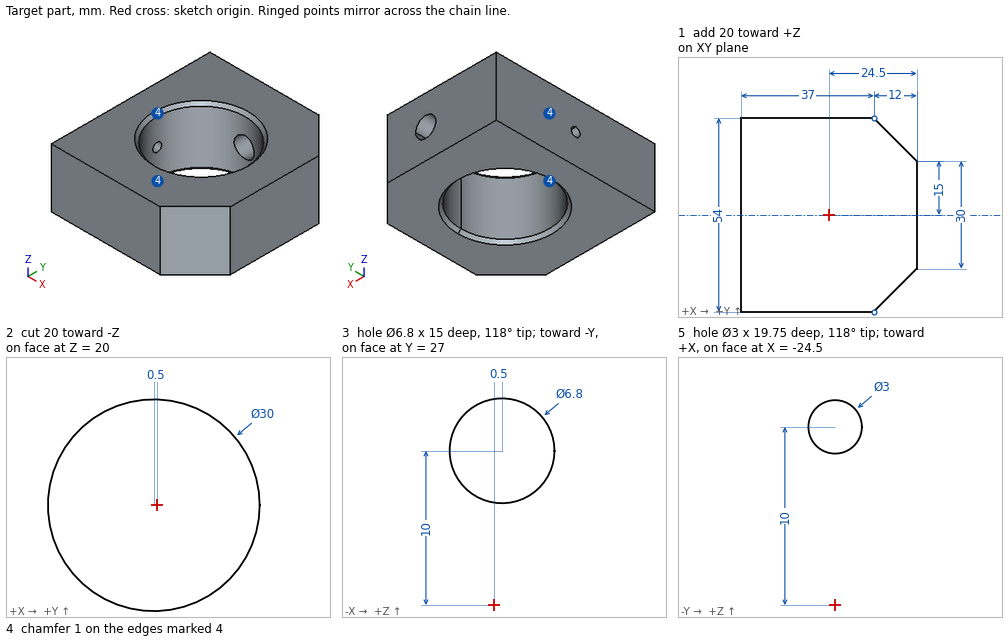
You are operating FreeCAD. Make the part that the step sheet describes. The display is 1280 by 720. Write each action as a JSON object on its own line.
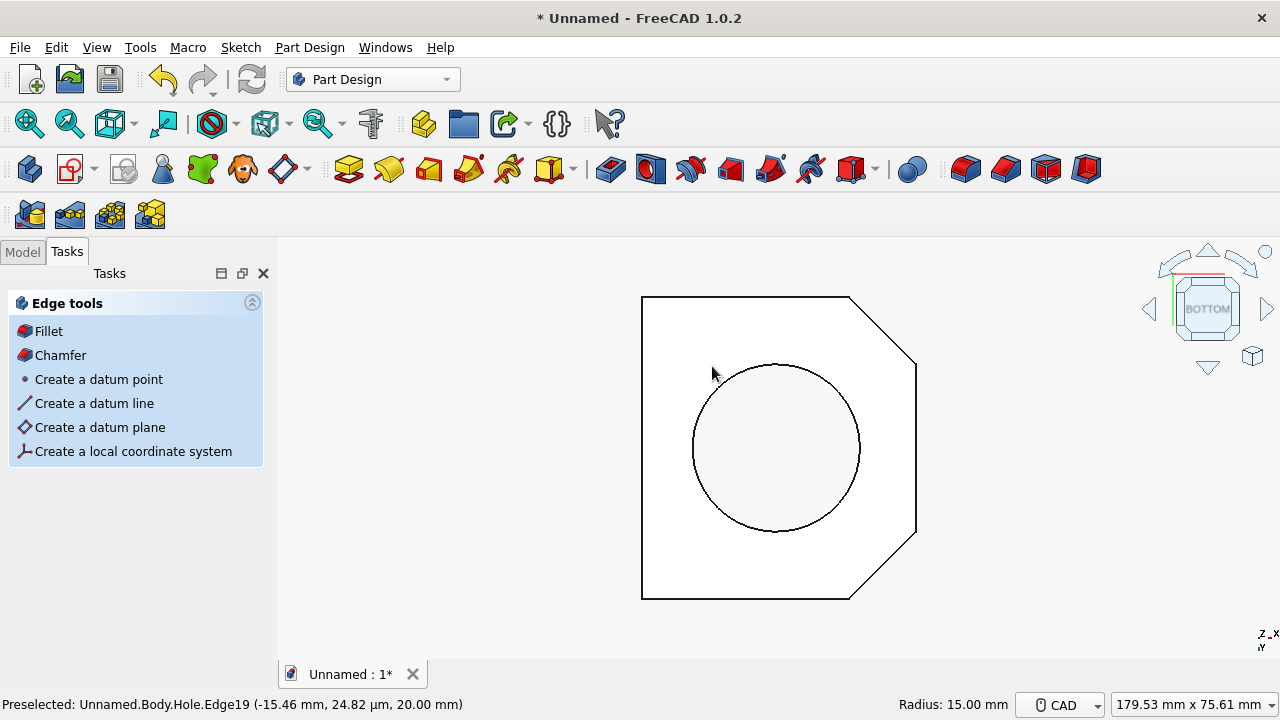
{"action": "left_click", "coordinate": [708, 496], "text": "ctrl"}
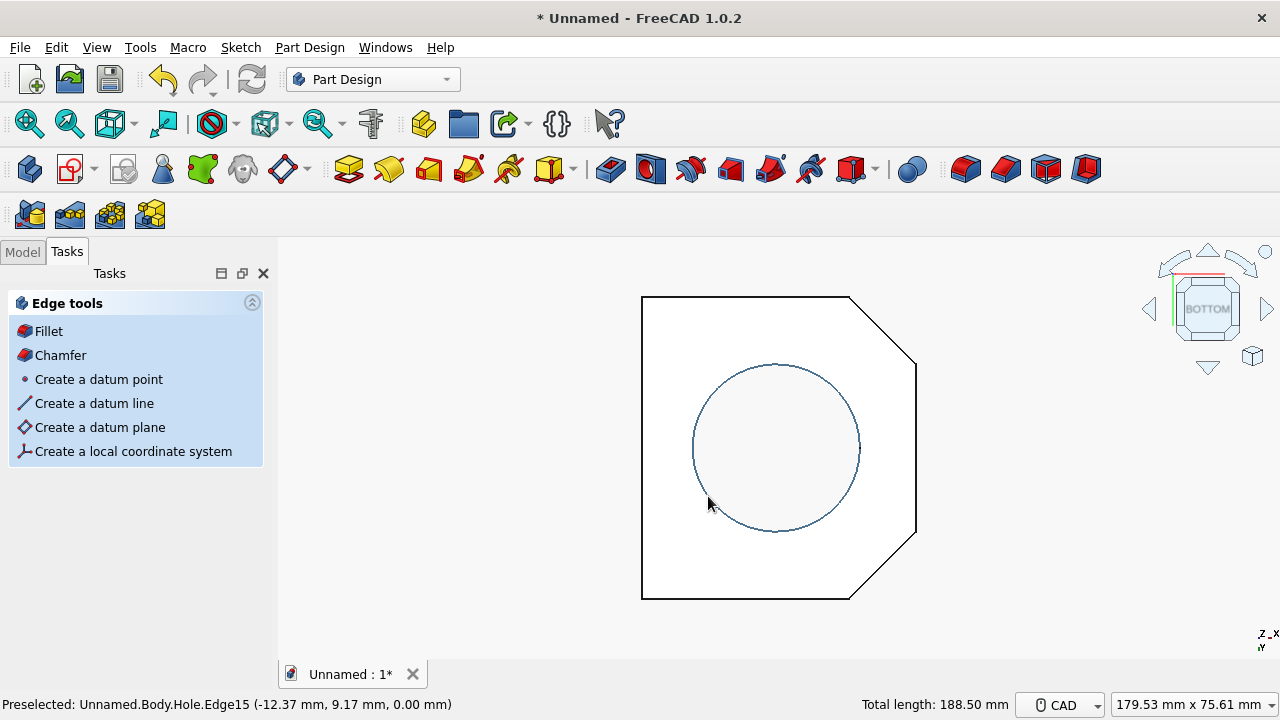
{"action": "left_click", "coordinate": [1006, 170]}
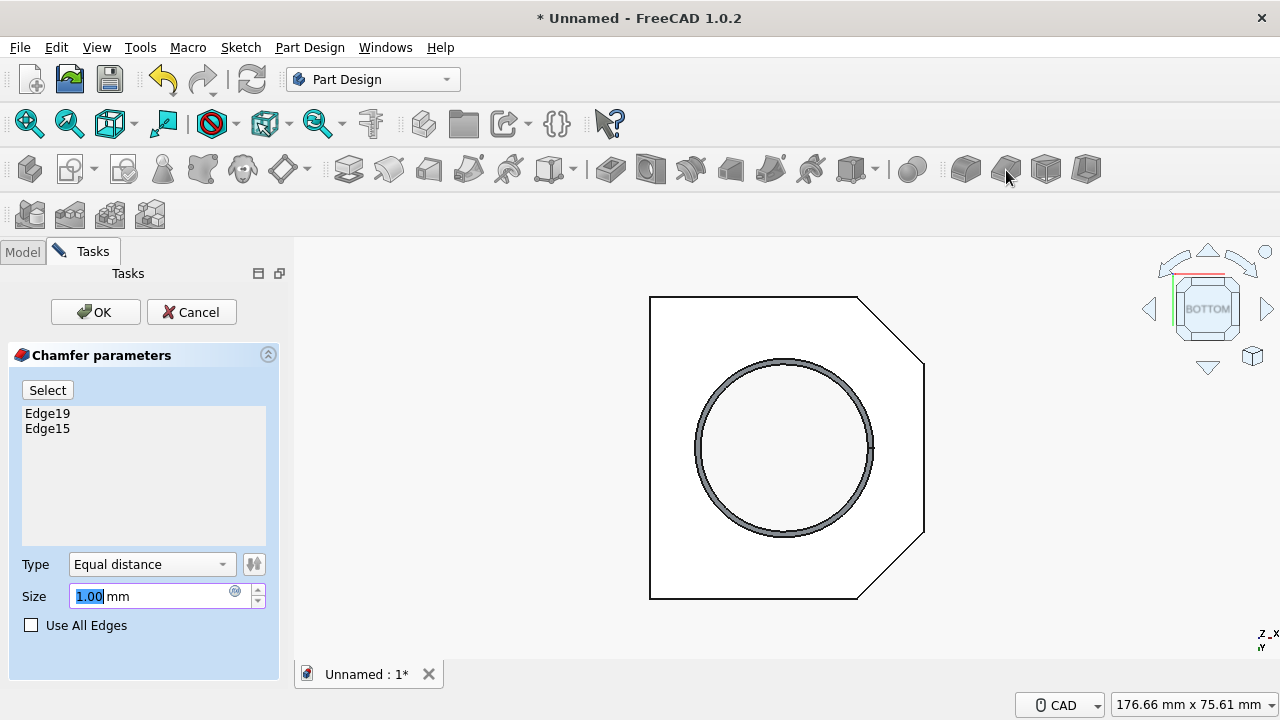
{"action": "type", "text": "1"}
{"action": "key", "text": "Tab"}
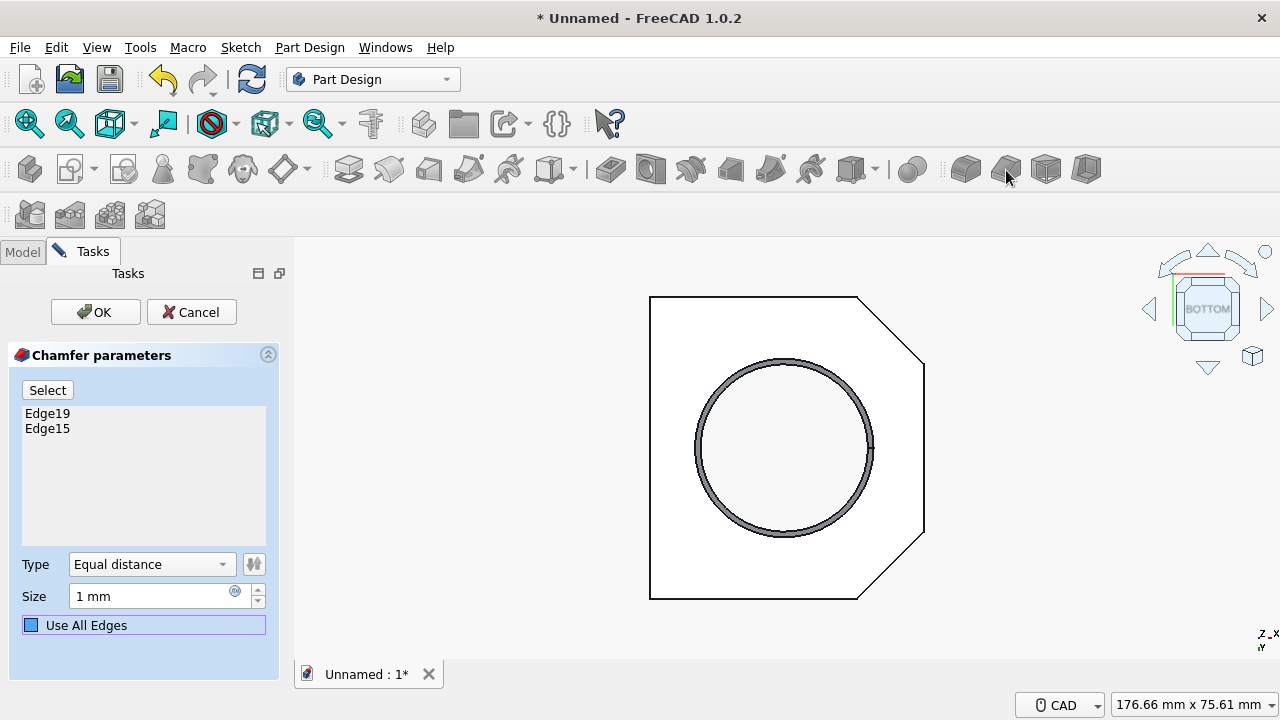
{"action": "left_click", "coordinate": [96, 312]}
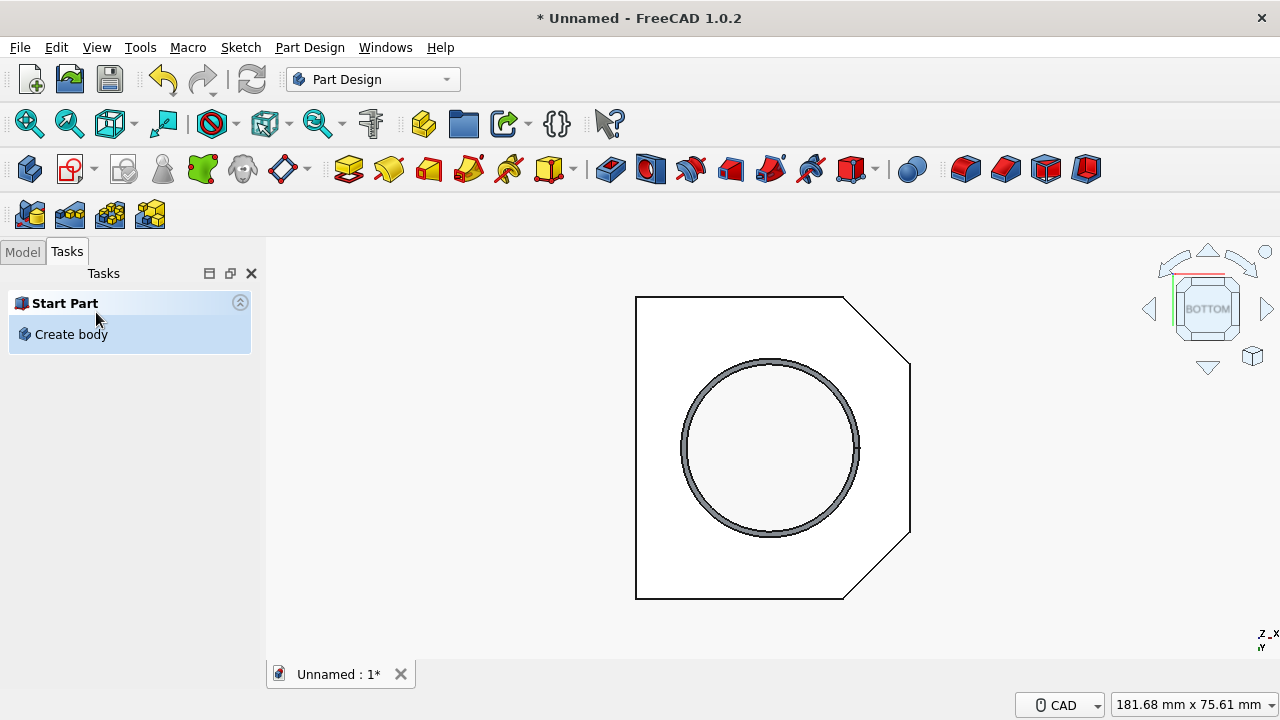
{"action": "key", "text": "6"}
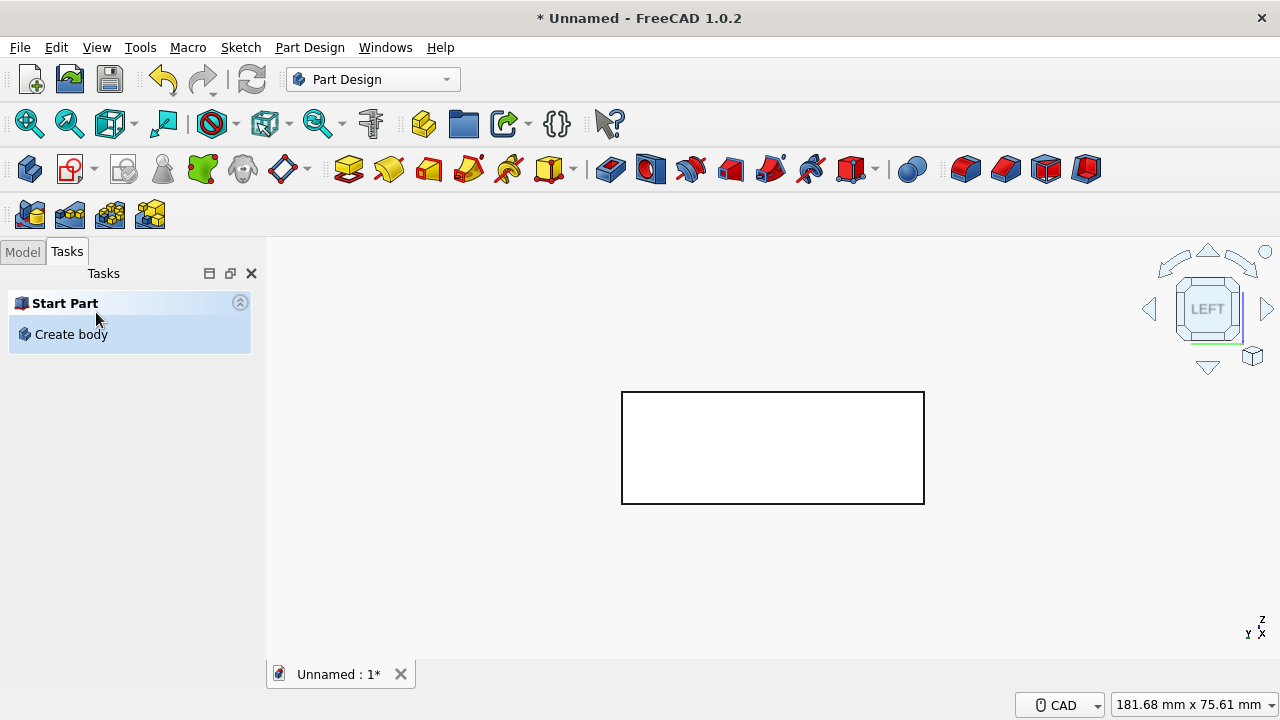
{"action": "left_click", "coordinate": [30, 124]}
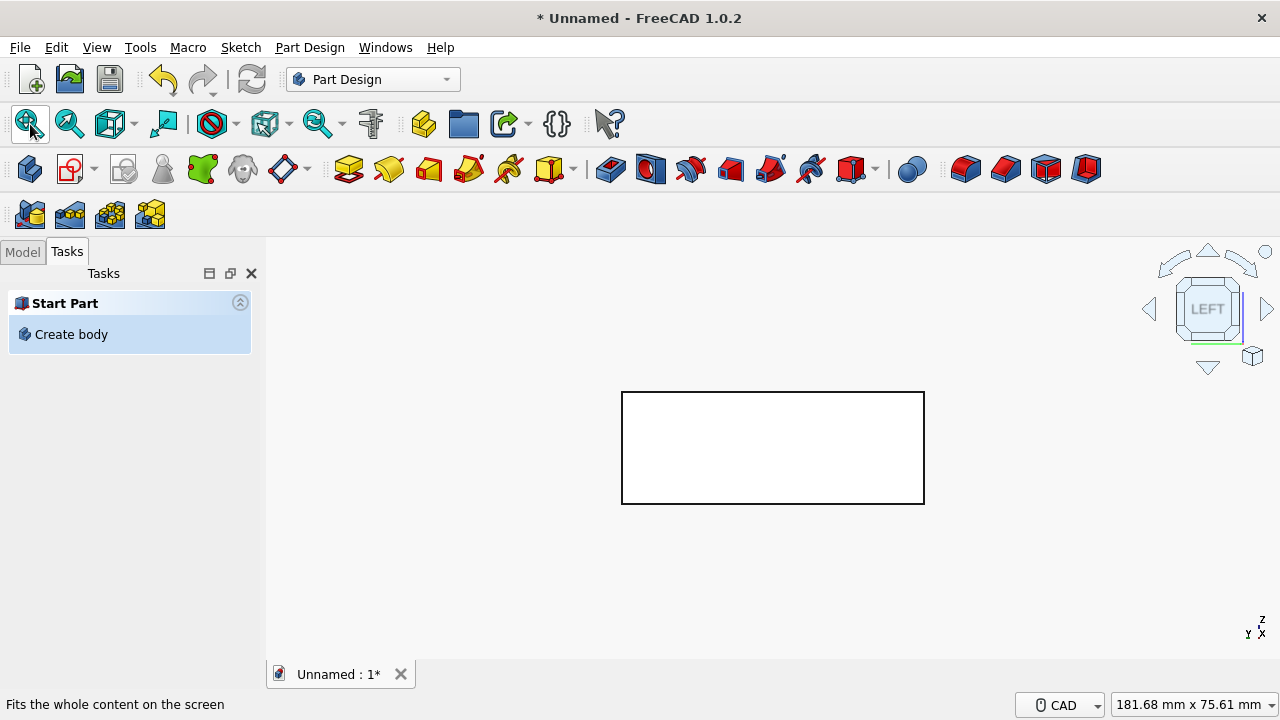
{"action": "left_click", "coordinate": [687, 447]}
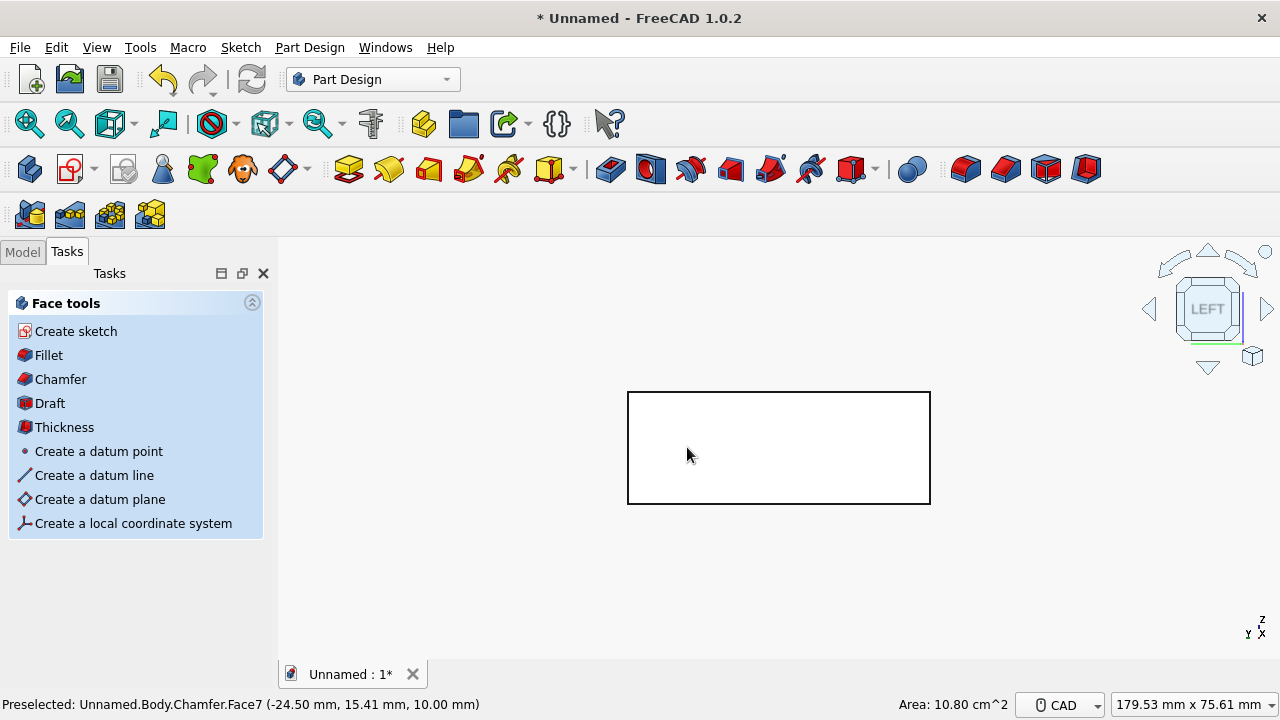
{"action": "left_click", "coordinate": [70, 170]}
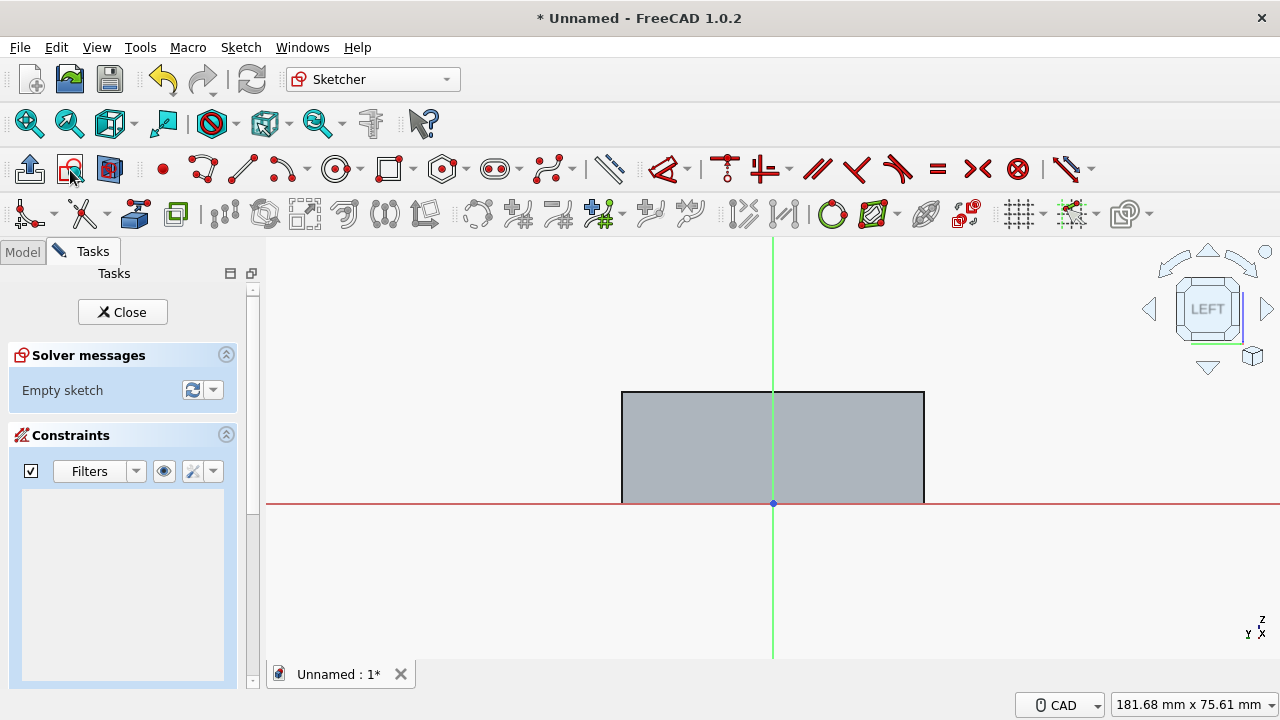
{"action": "scroll", "coordinate": [777, 448], "scroll_direction": "up", "scroll_amount": 14}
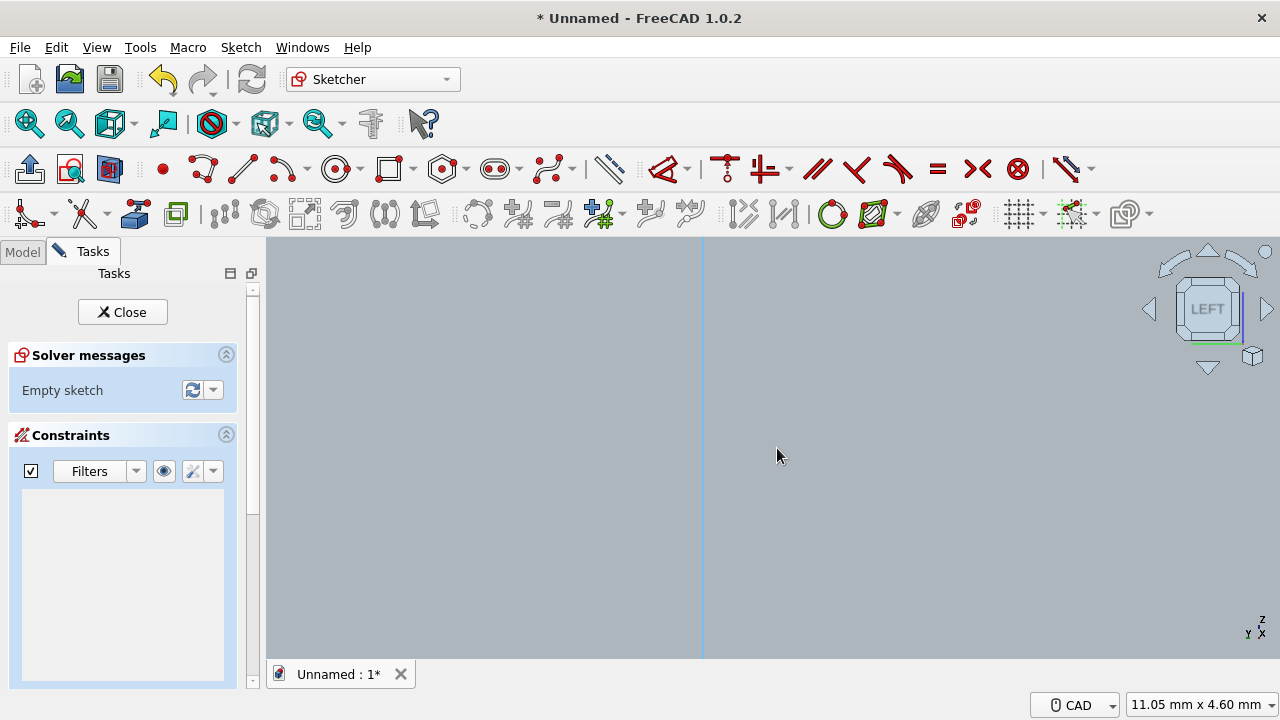
{"action": "key", "text": "g c"}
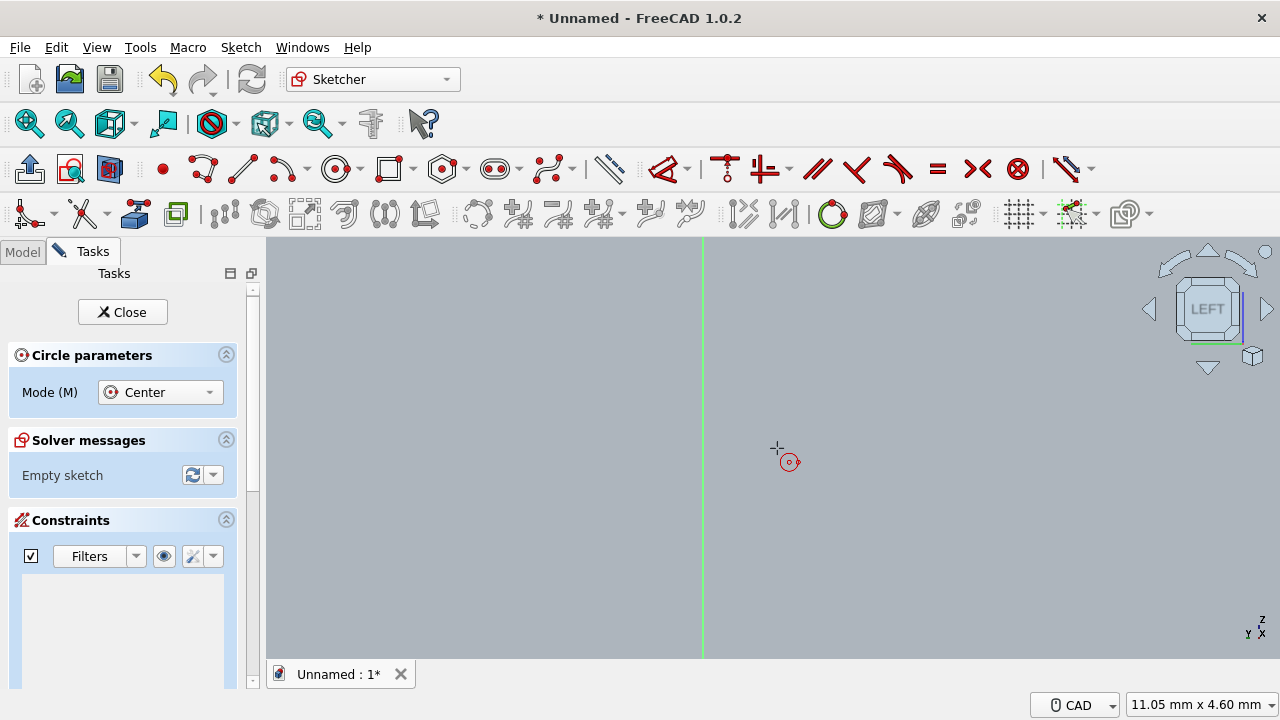
{"action": "left_click", "coordinate": [703, 440]}
{"action": "left_click", "coordinate": [801, 343]}
{"action": "key", "text": "Escape"}